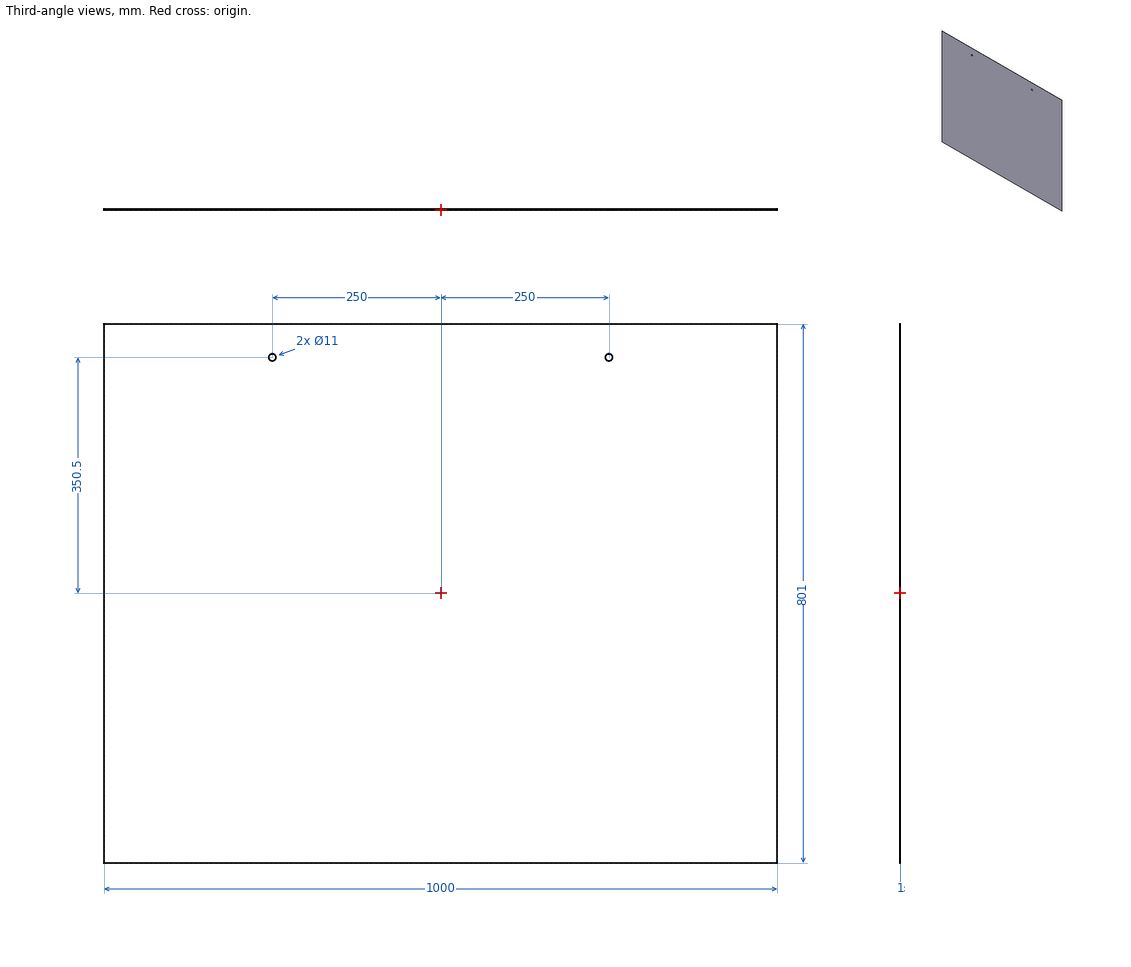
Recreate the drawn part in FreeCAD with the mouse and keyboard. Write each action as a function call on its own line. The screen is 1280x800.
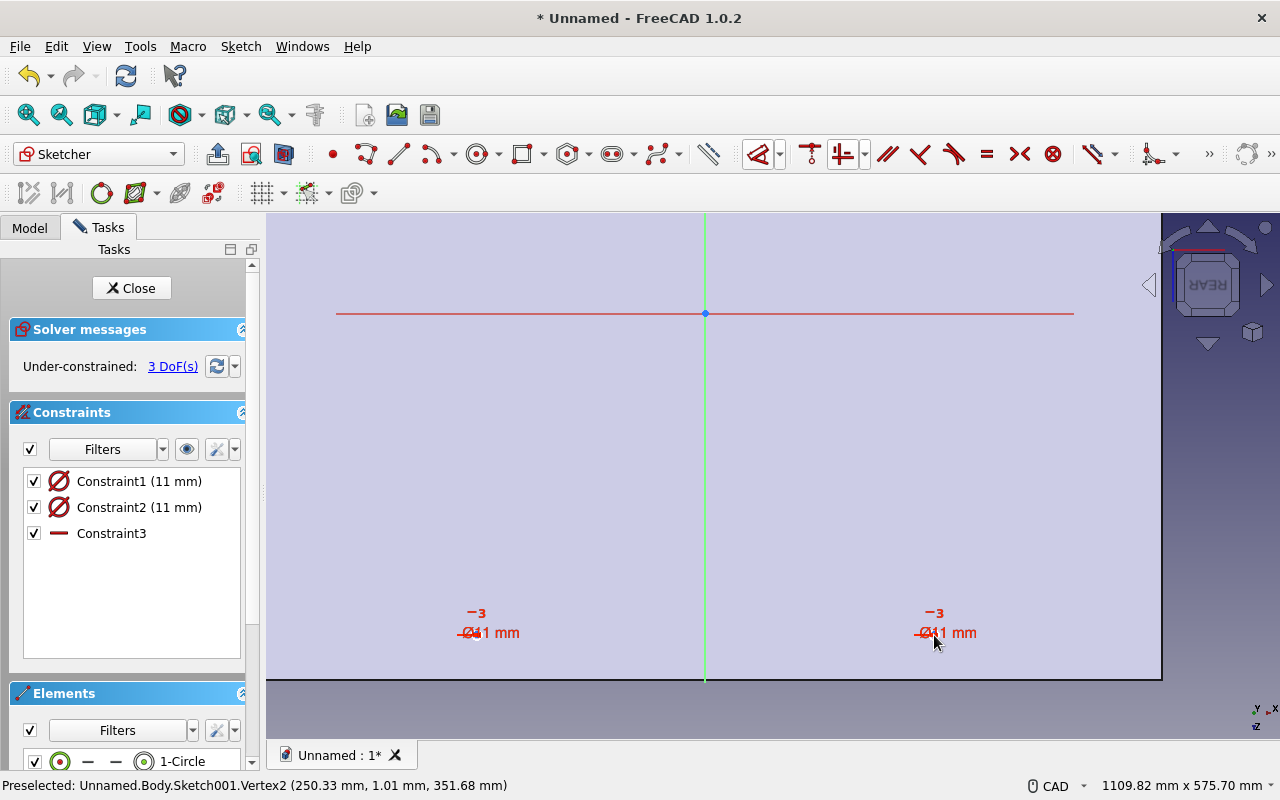
click(477, 635)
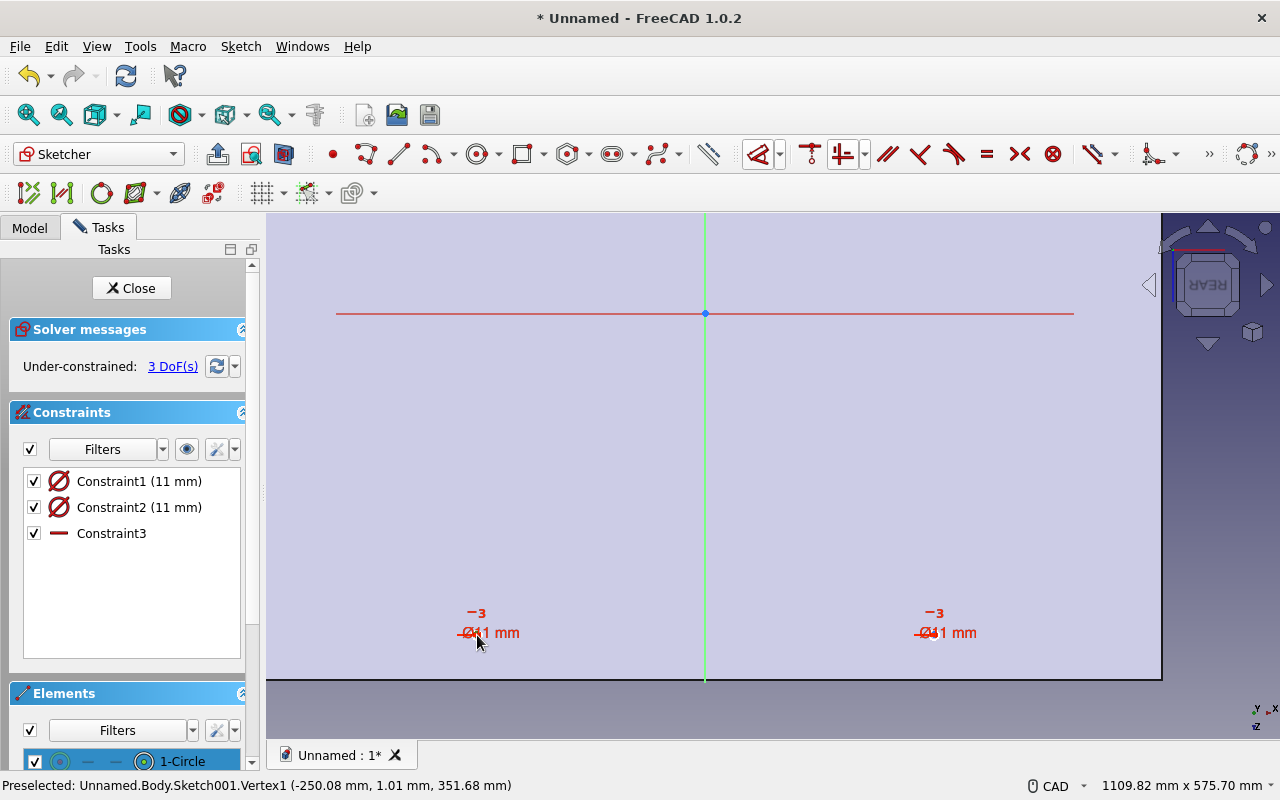
key(l)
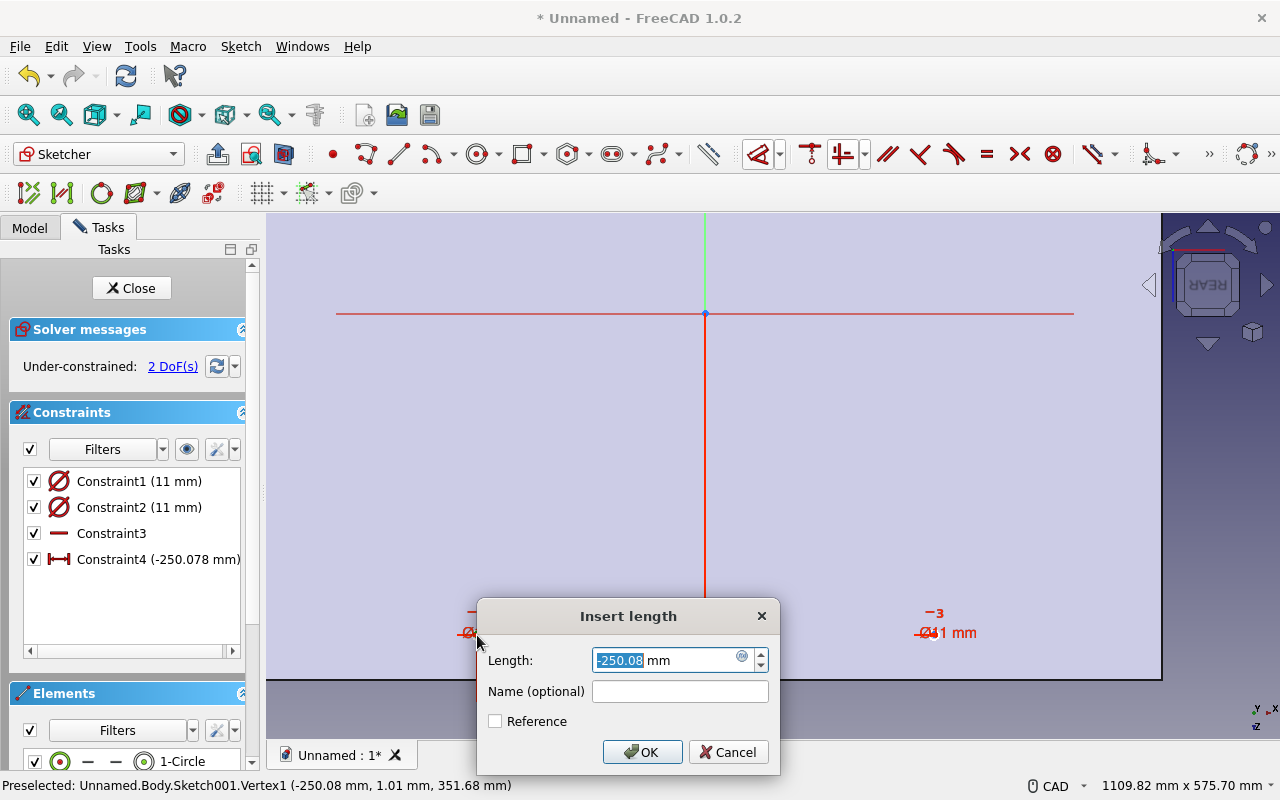
text(-250)
key(Return)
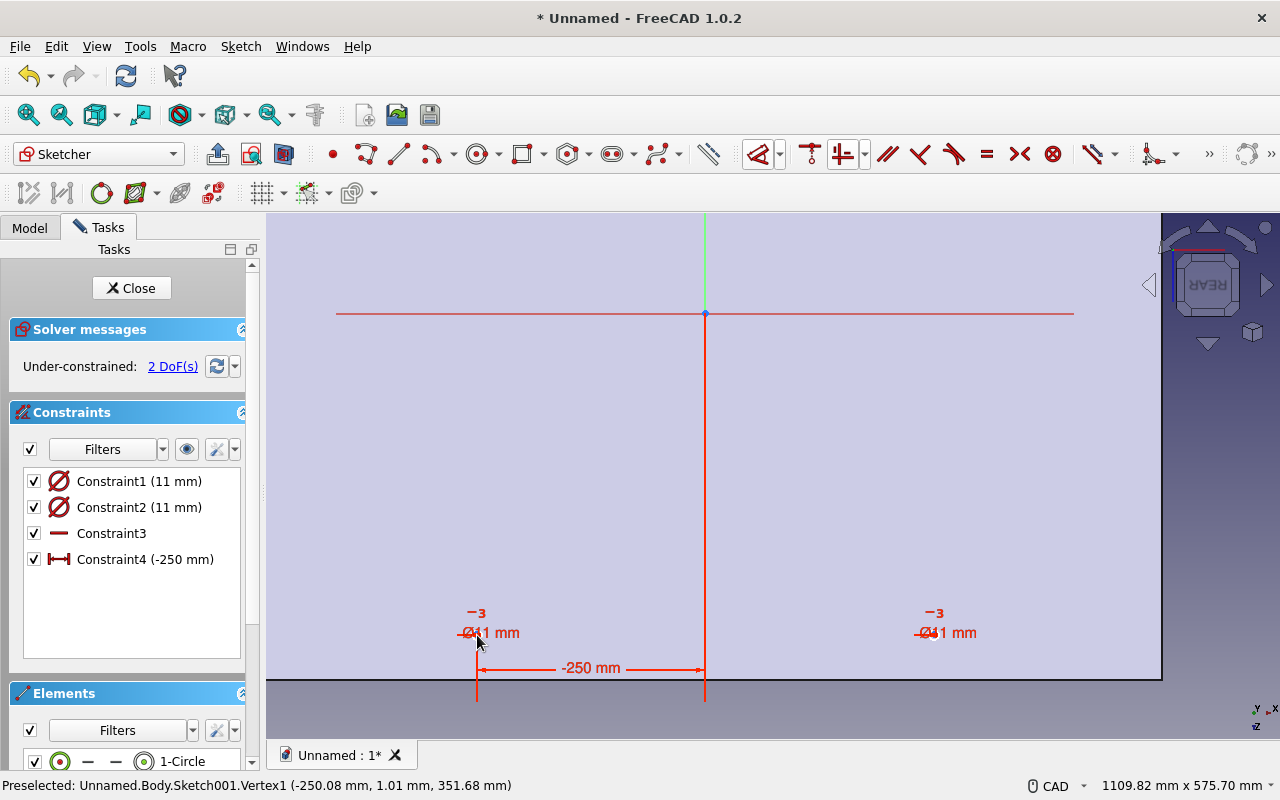
click(934, 635)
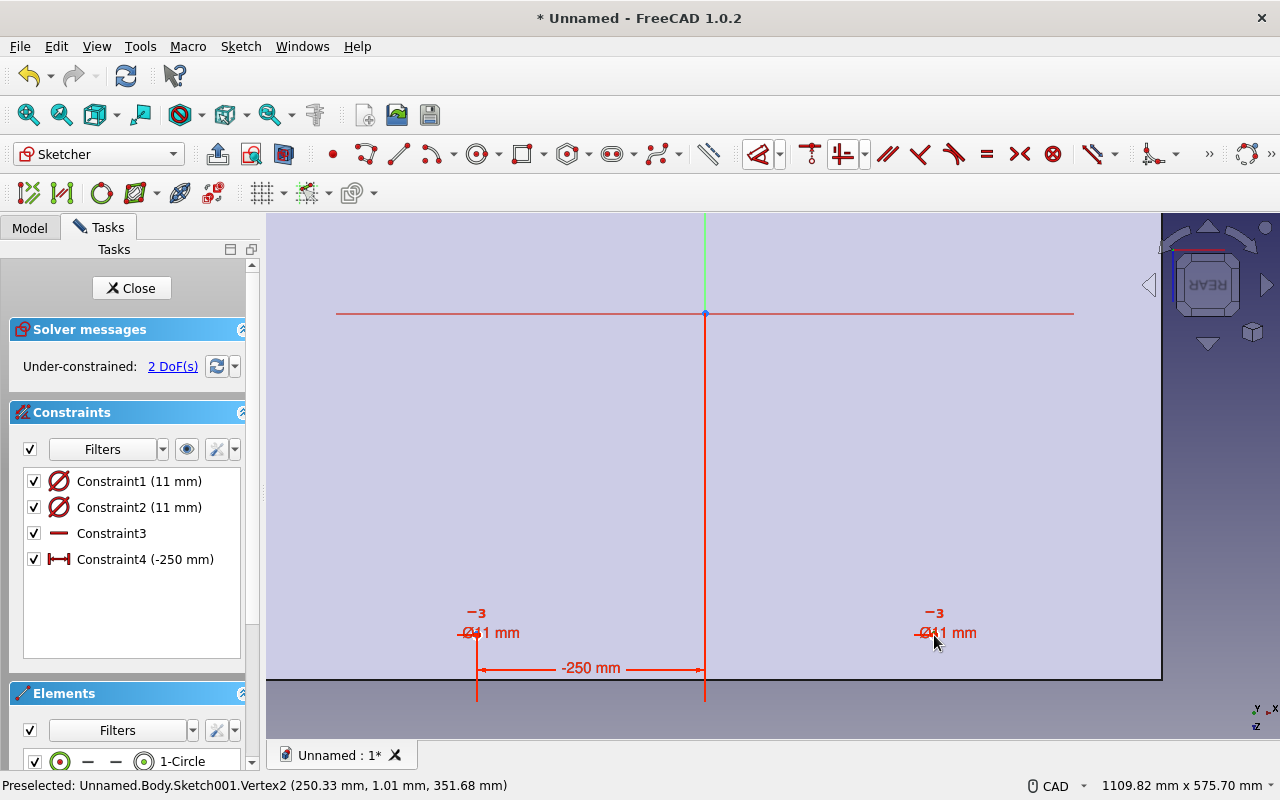
click(780, 154)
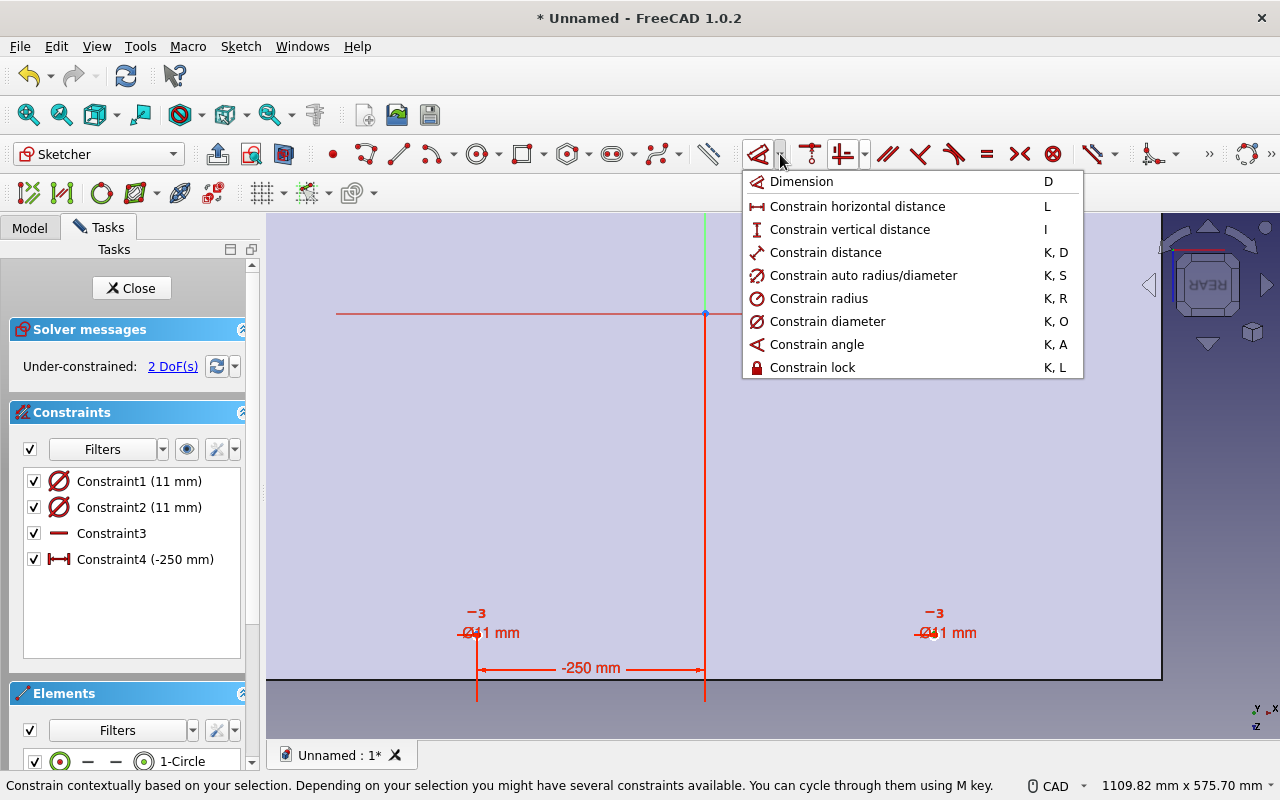
click(913, 206)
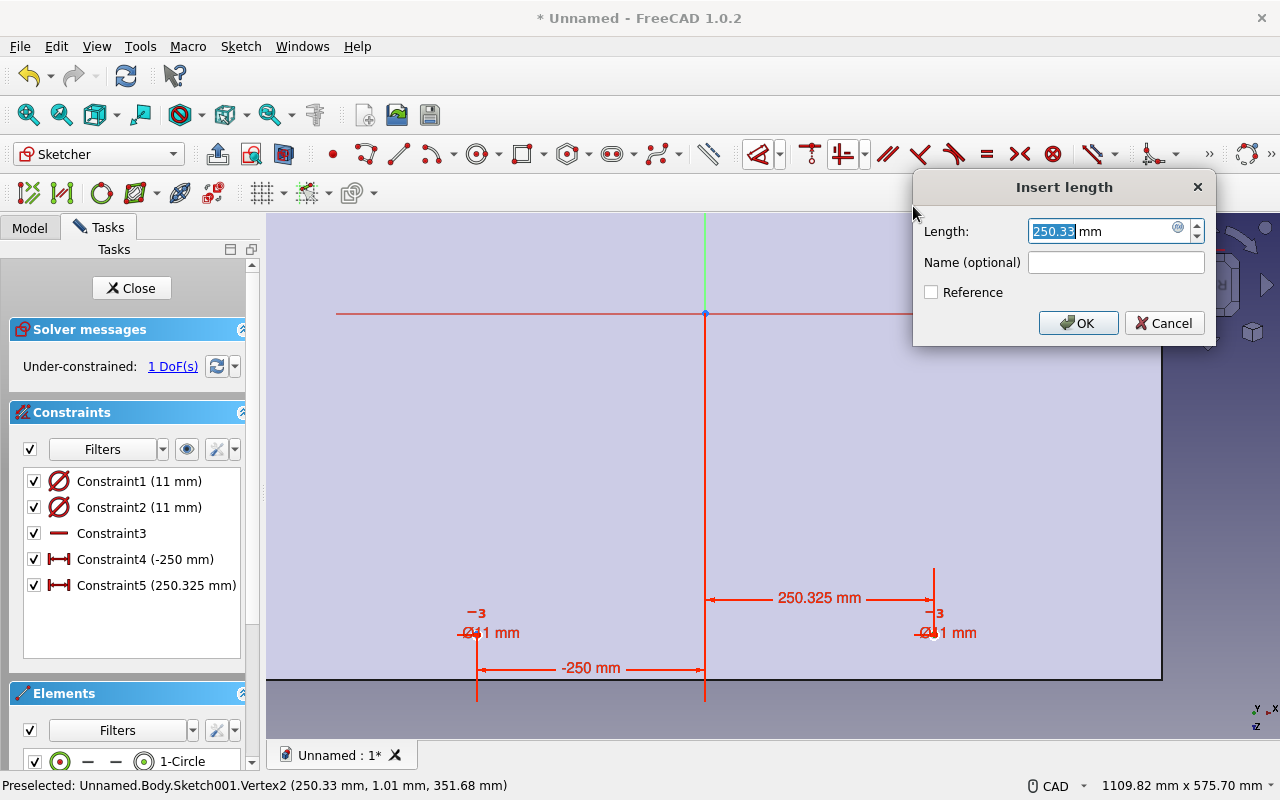
text(250)
key(Return)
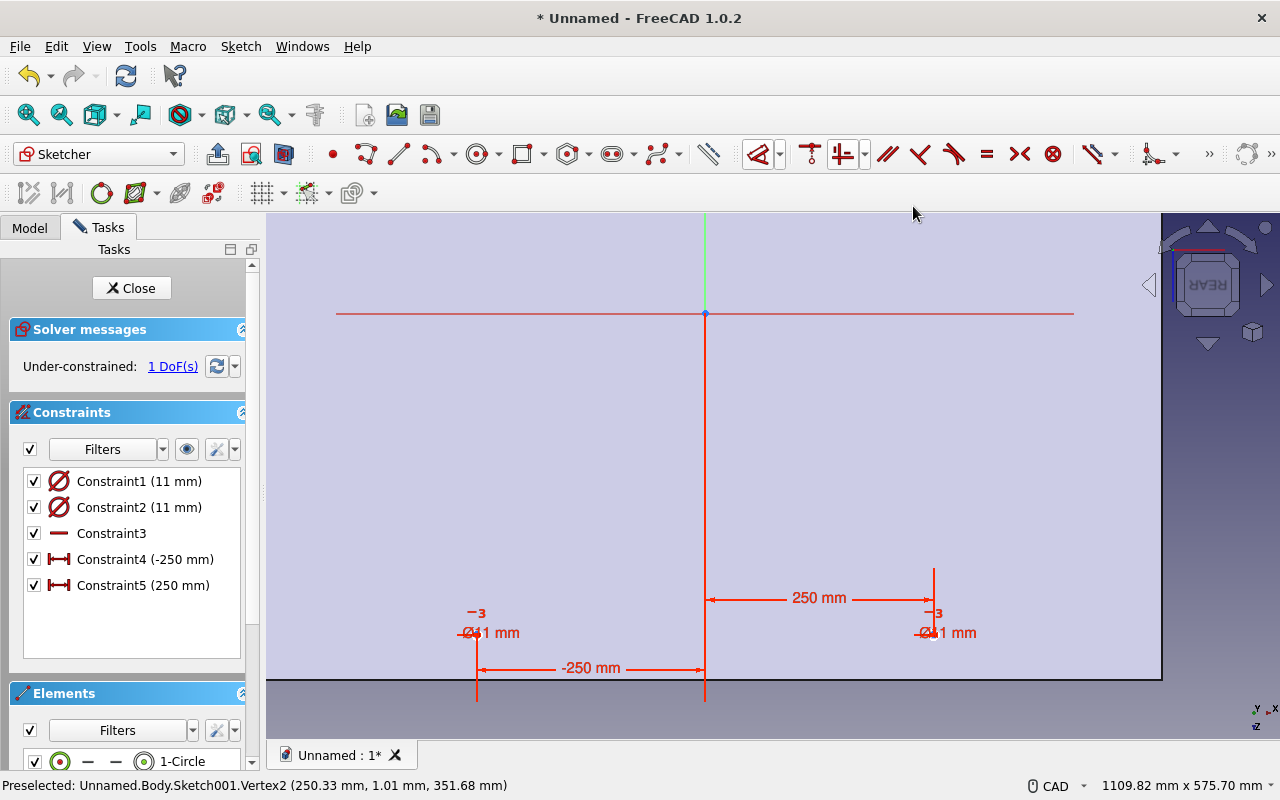
click(477, 635)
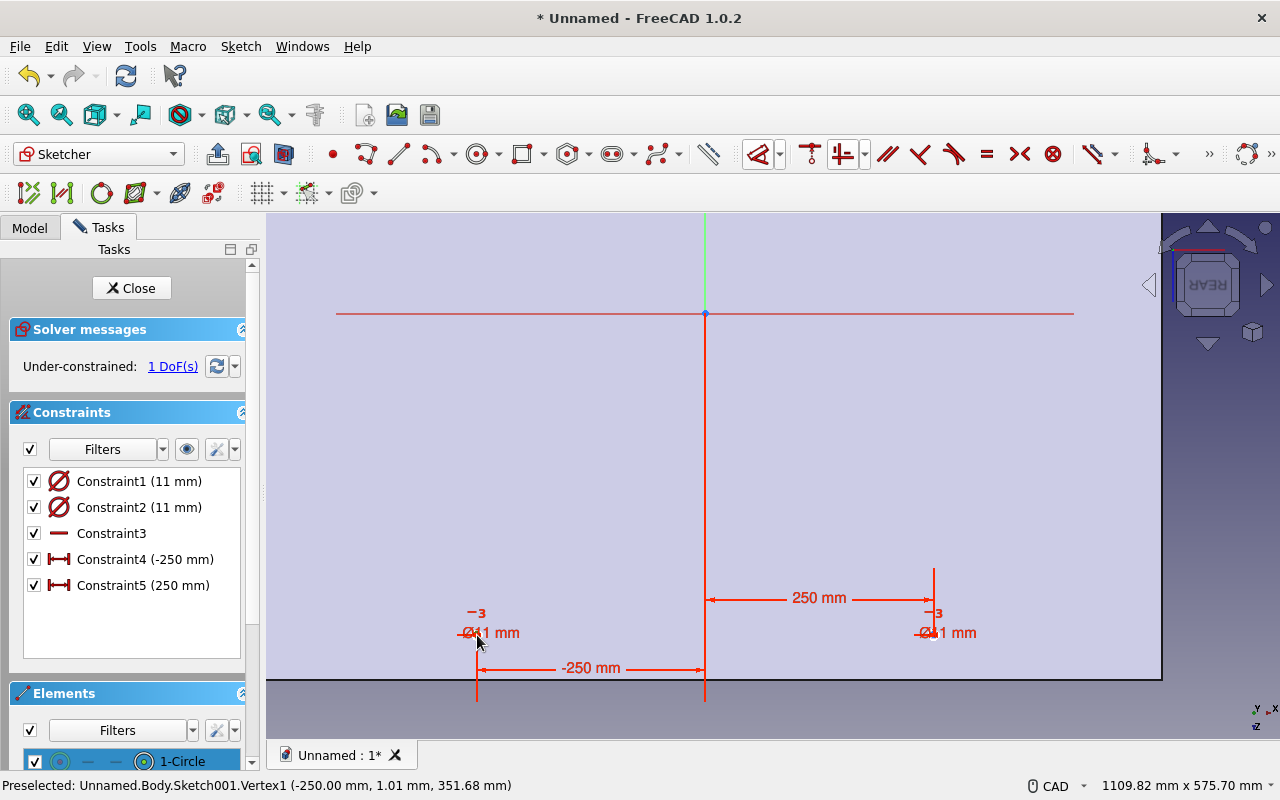
key(i)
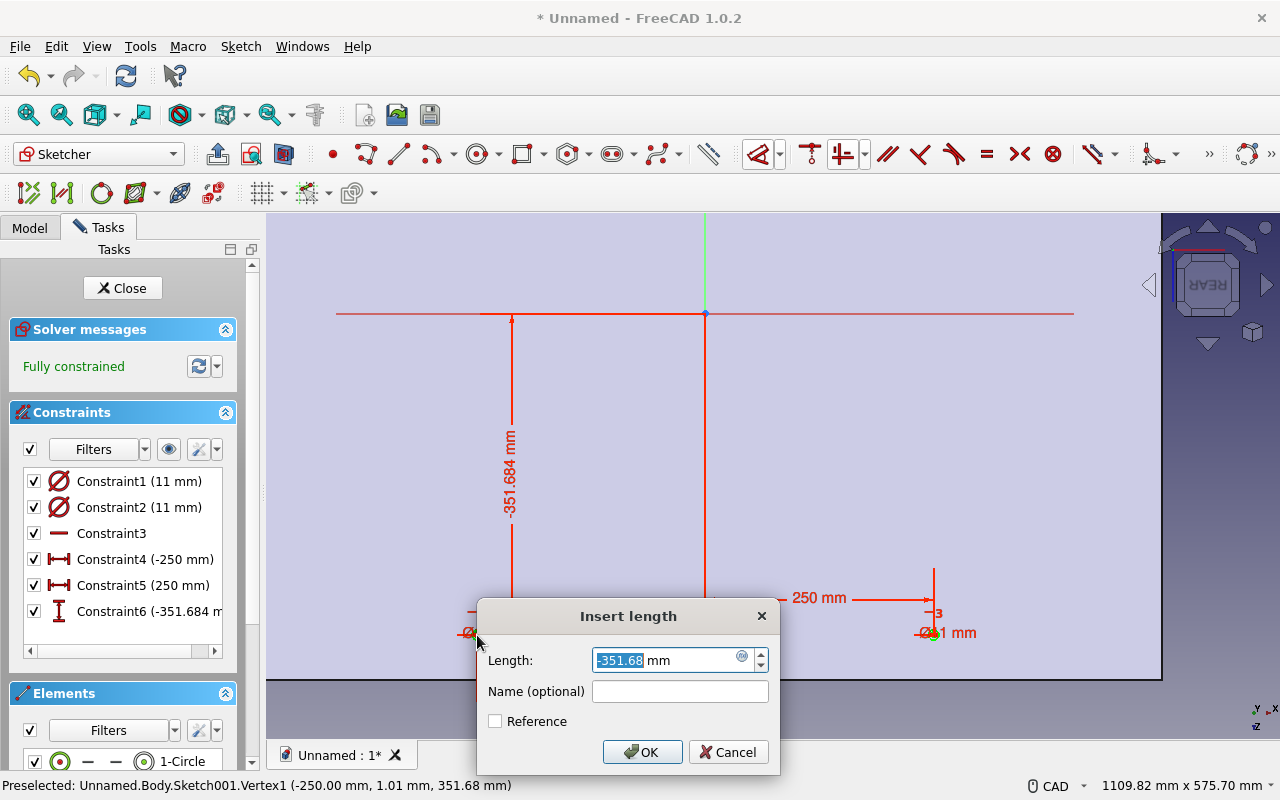
text(-350.5)
key(Return)